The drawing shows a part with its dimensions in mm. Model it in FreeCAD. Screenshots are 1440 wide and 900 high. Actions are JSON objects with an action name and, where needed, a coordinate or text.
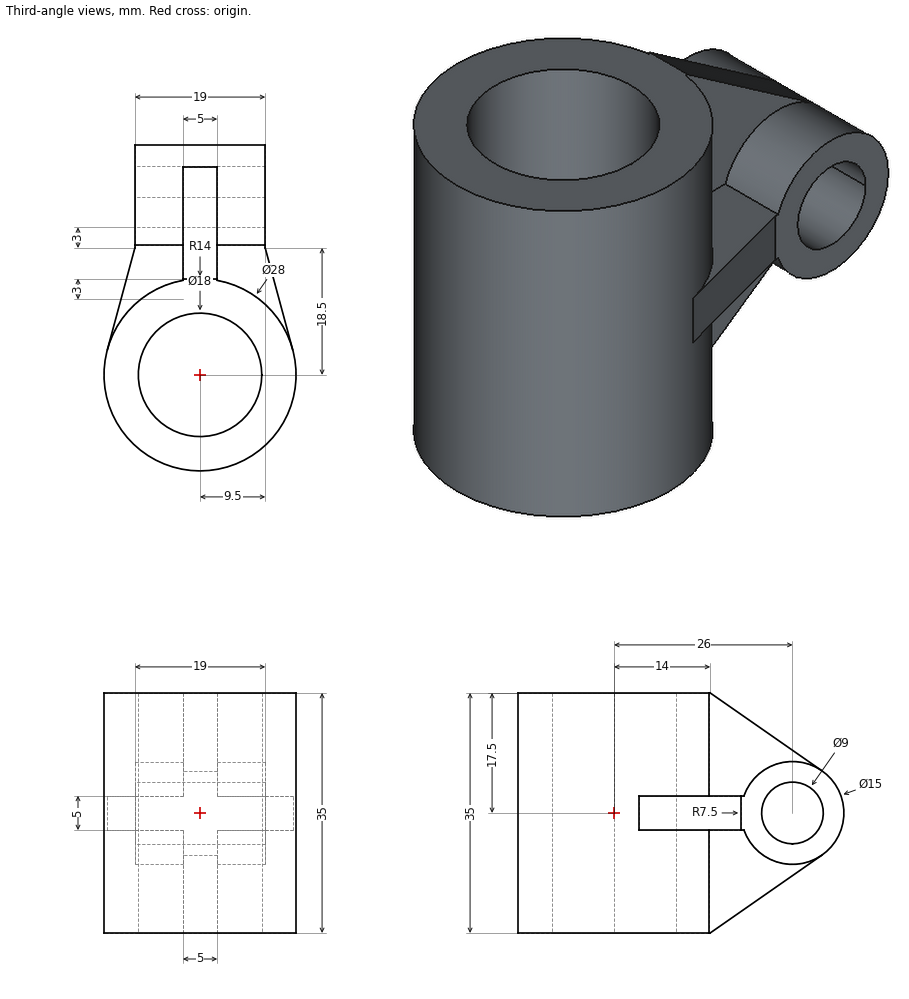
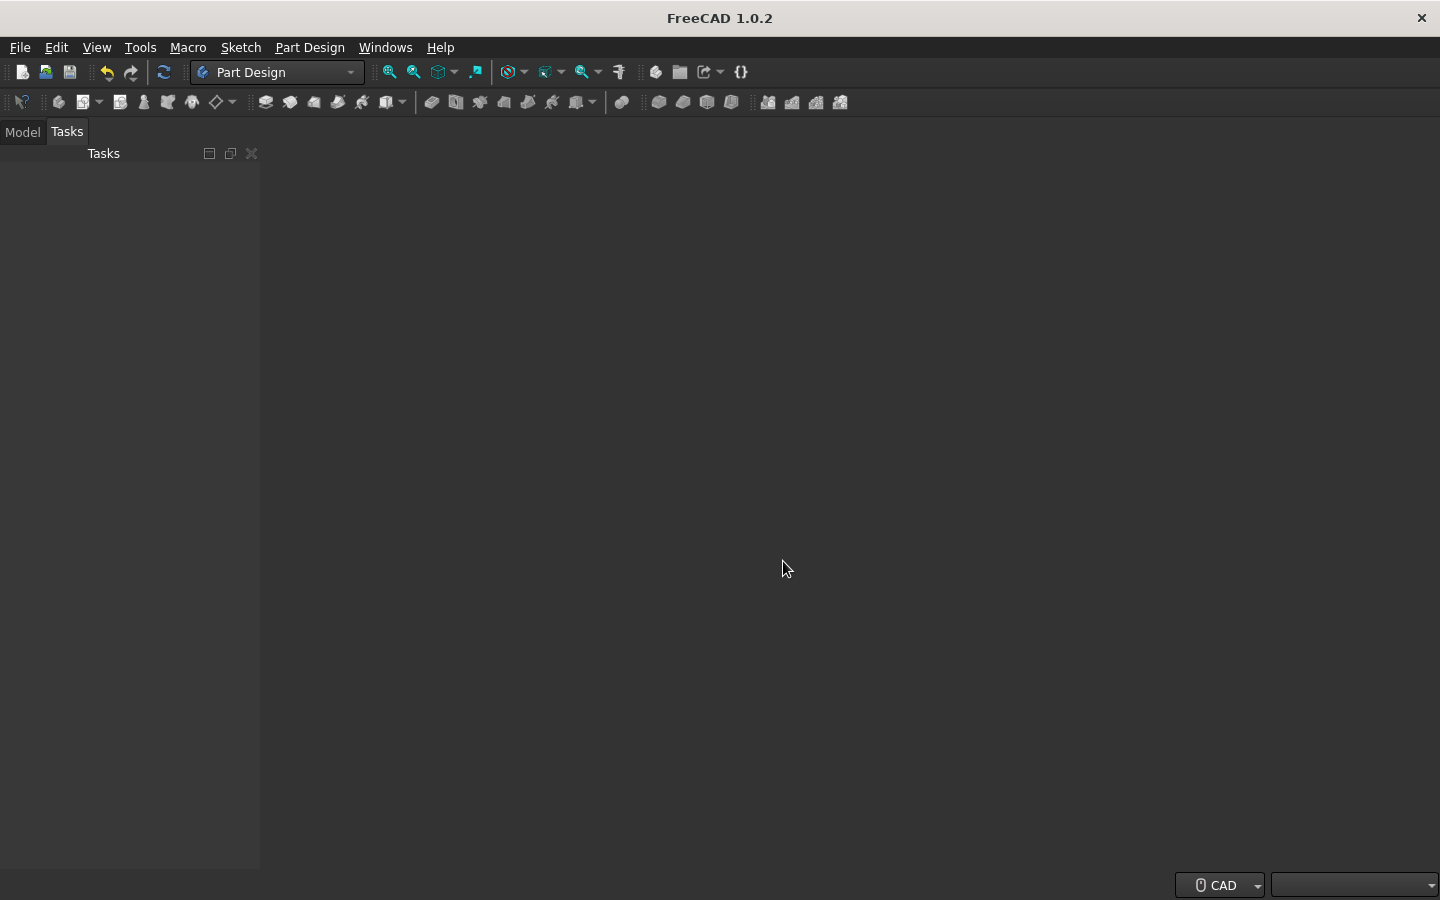
{"action": "key", "text": "ctrl+n"}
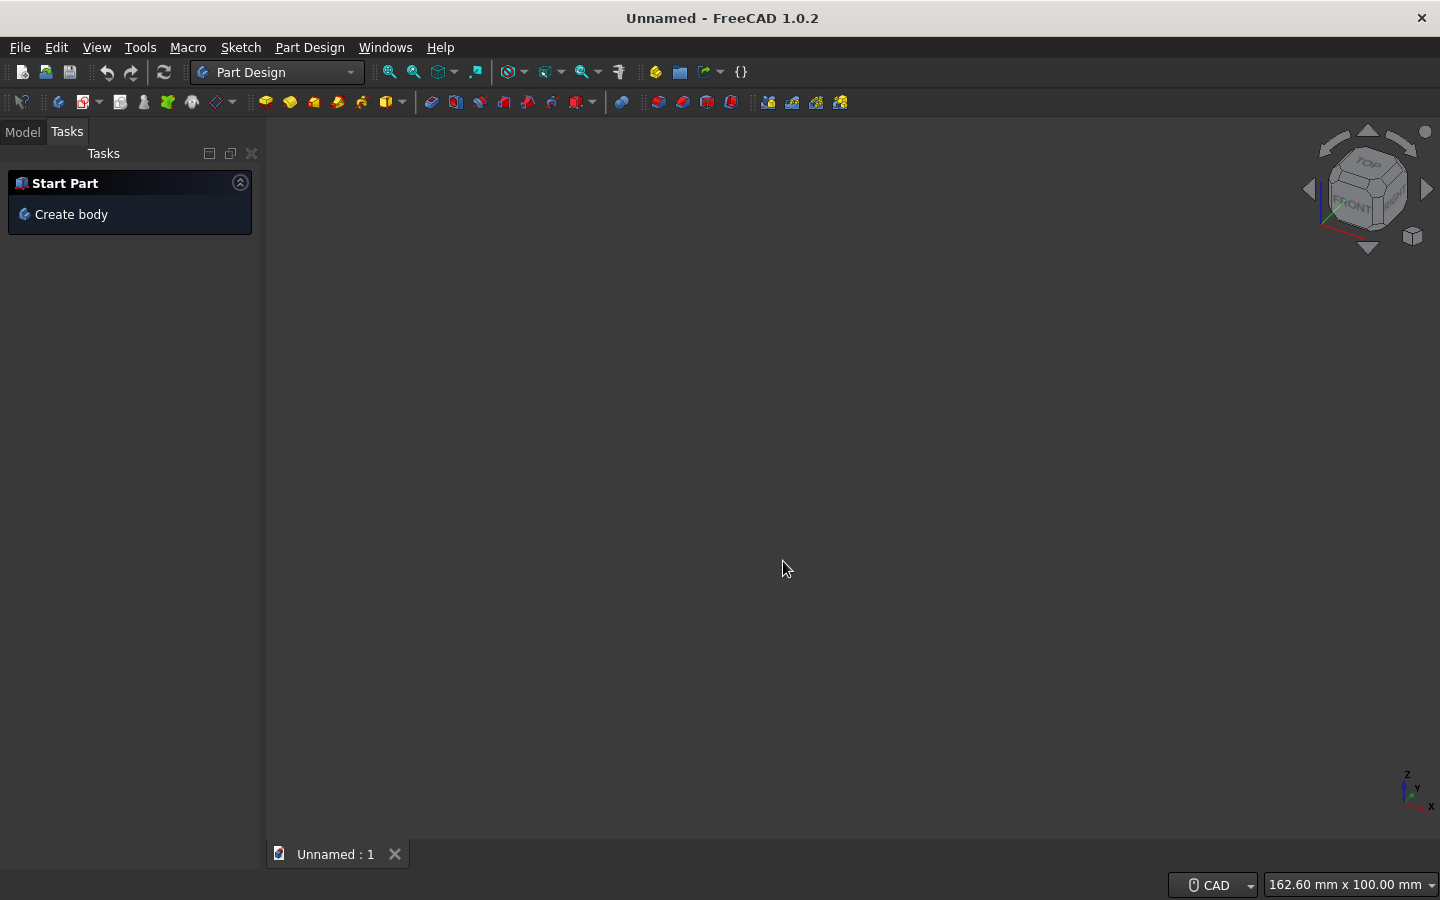
{"action": "left_click", "coordinate": [84, 102]}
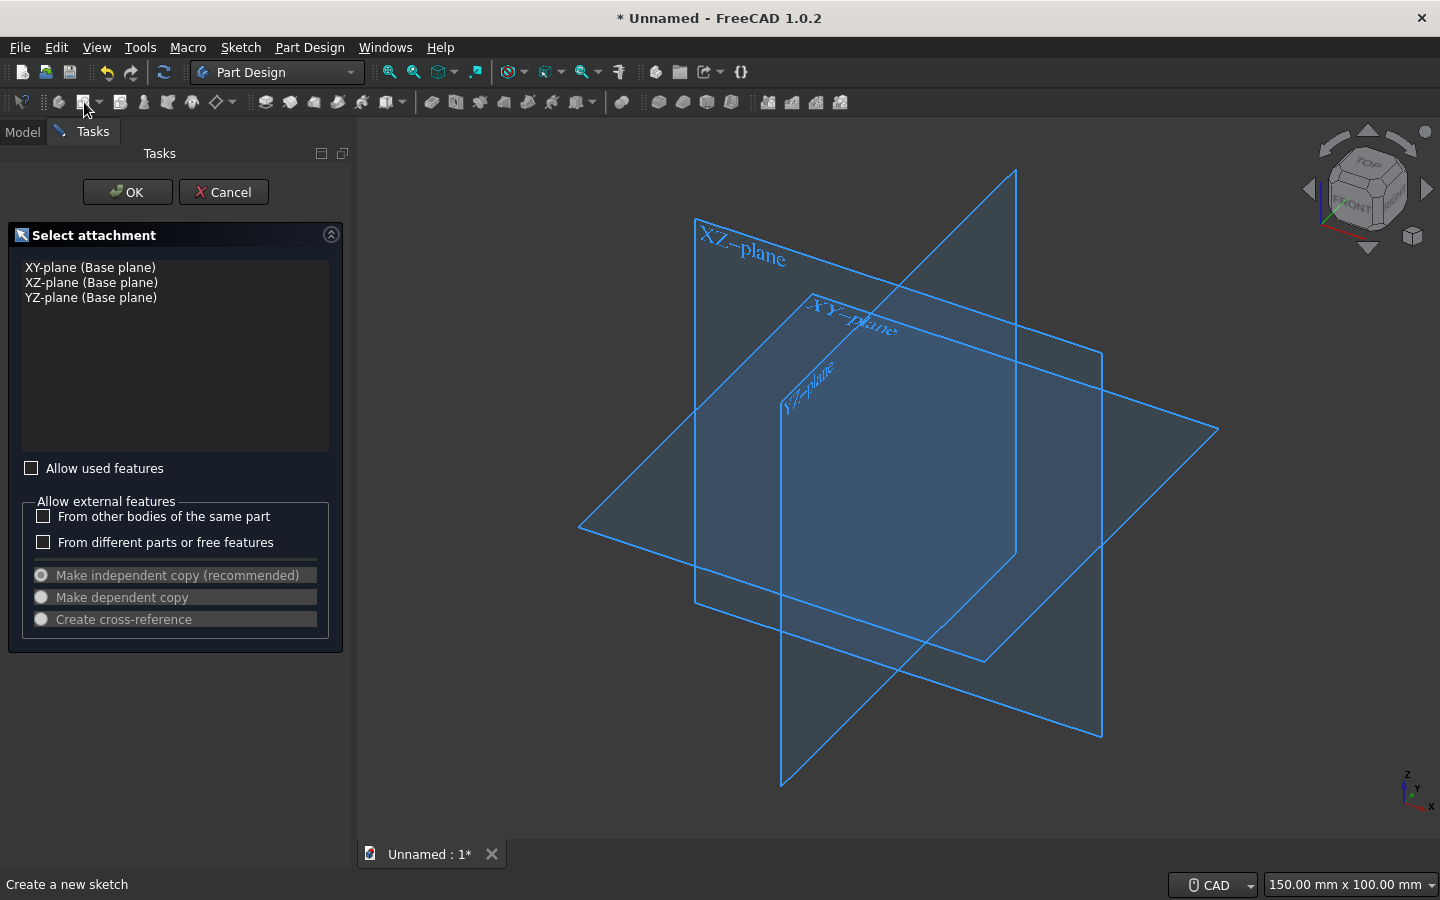
{"action": "left_click", "coordinate": [82, 268]}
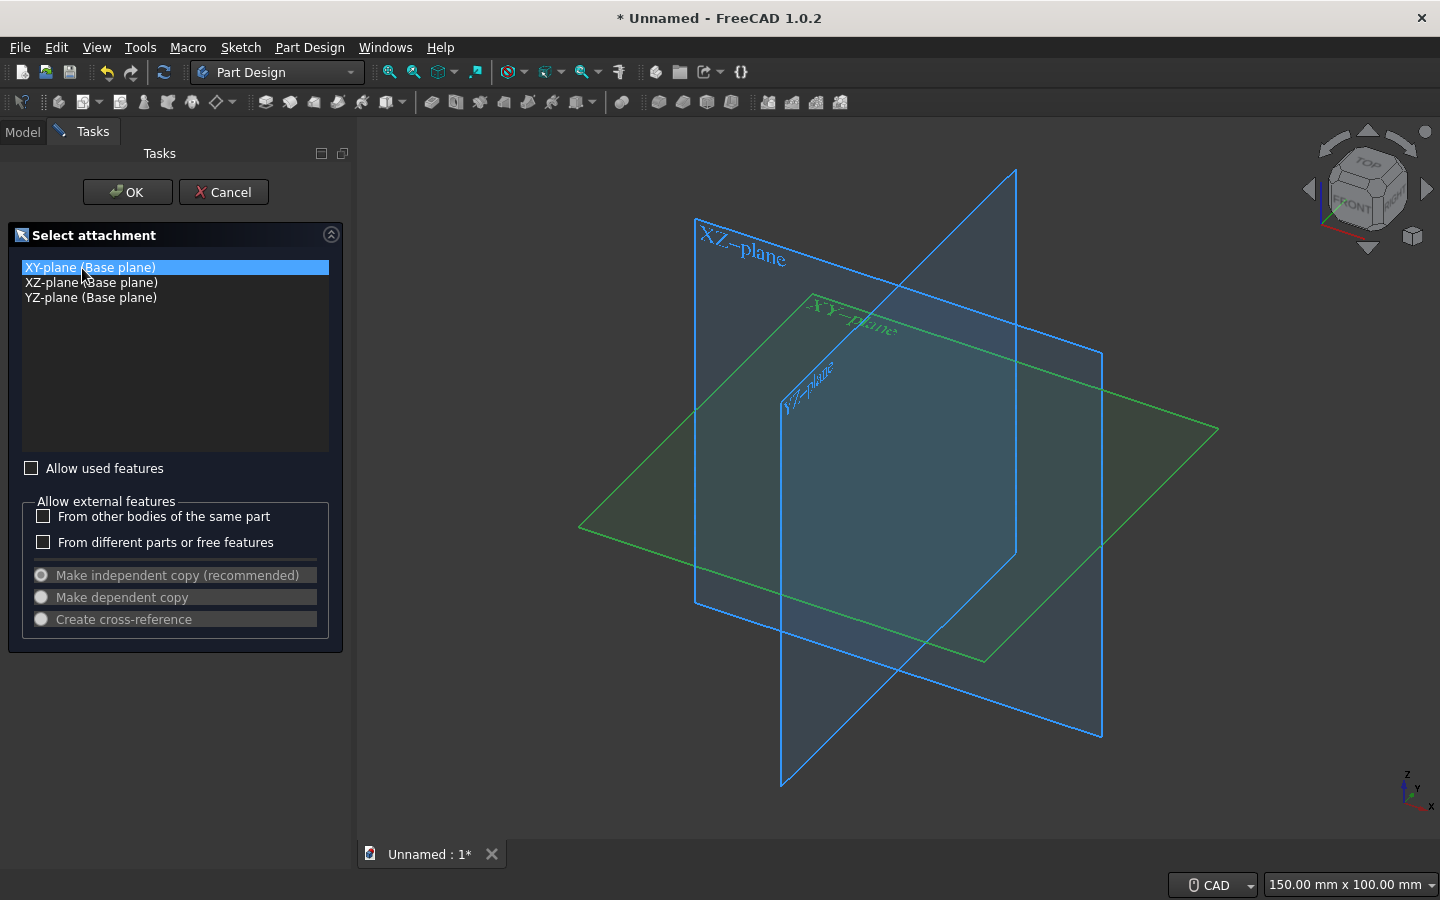
{"action": "left_click", "coordinate": [128, 192]}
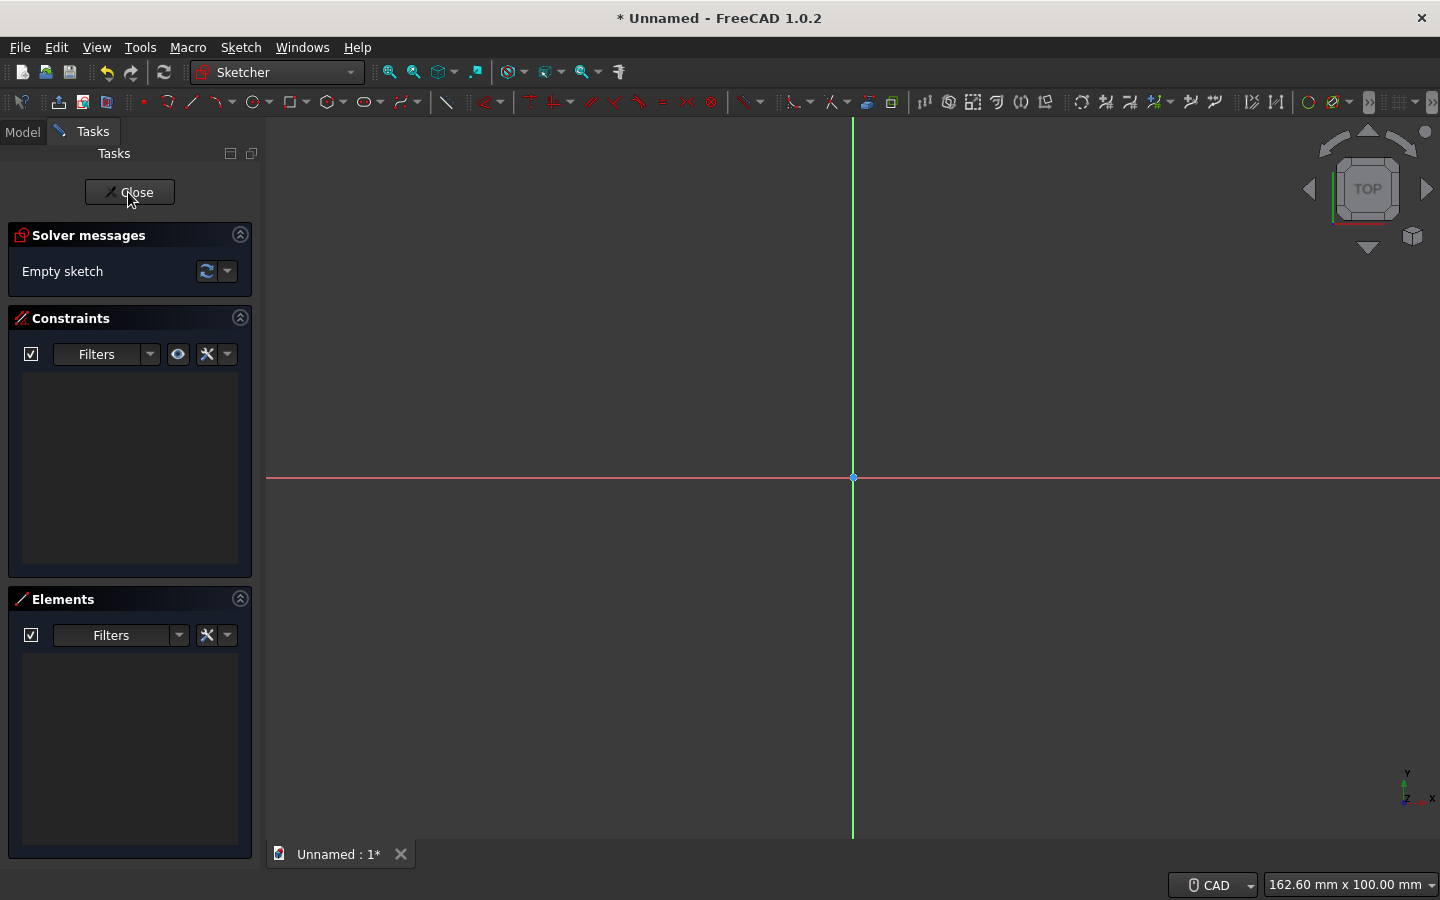
{"action": "scroll", "coordinate": [909, 478], "scroll_direction": "up", "scroll_amount": 4}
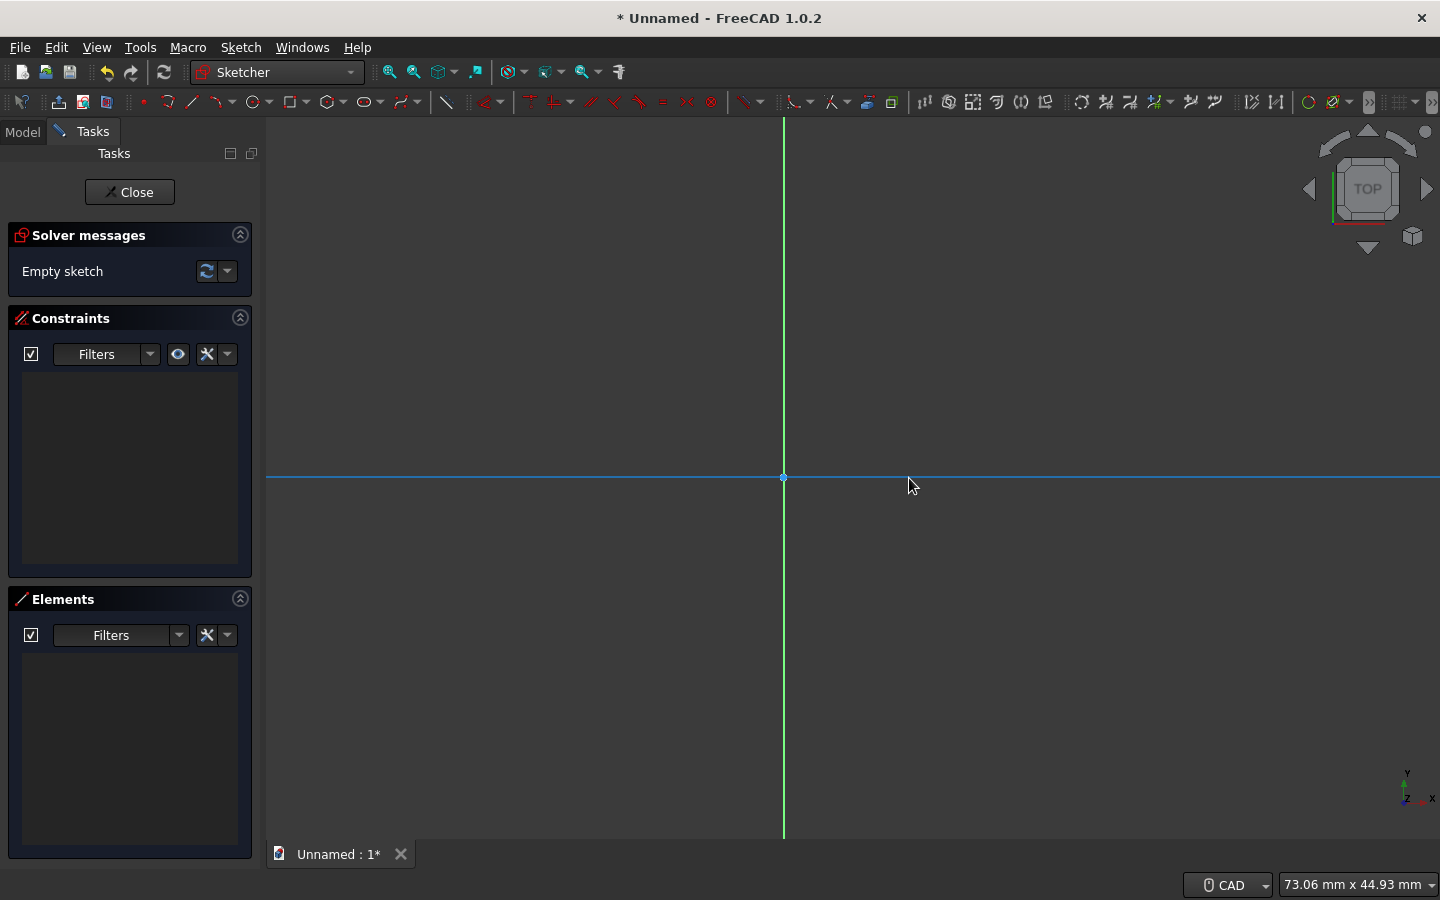
{"action": "key", "text": "g c"}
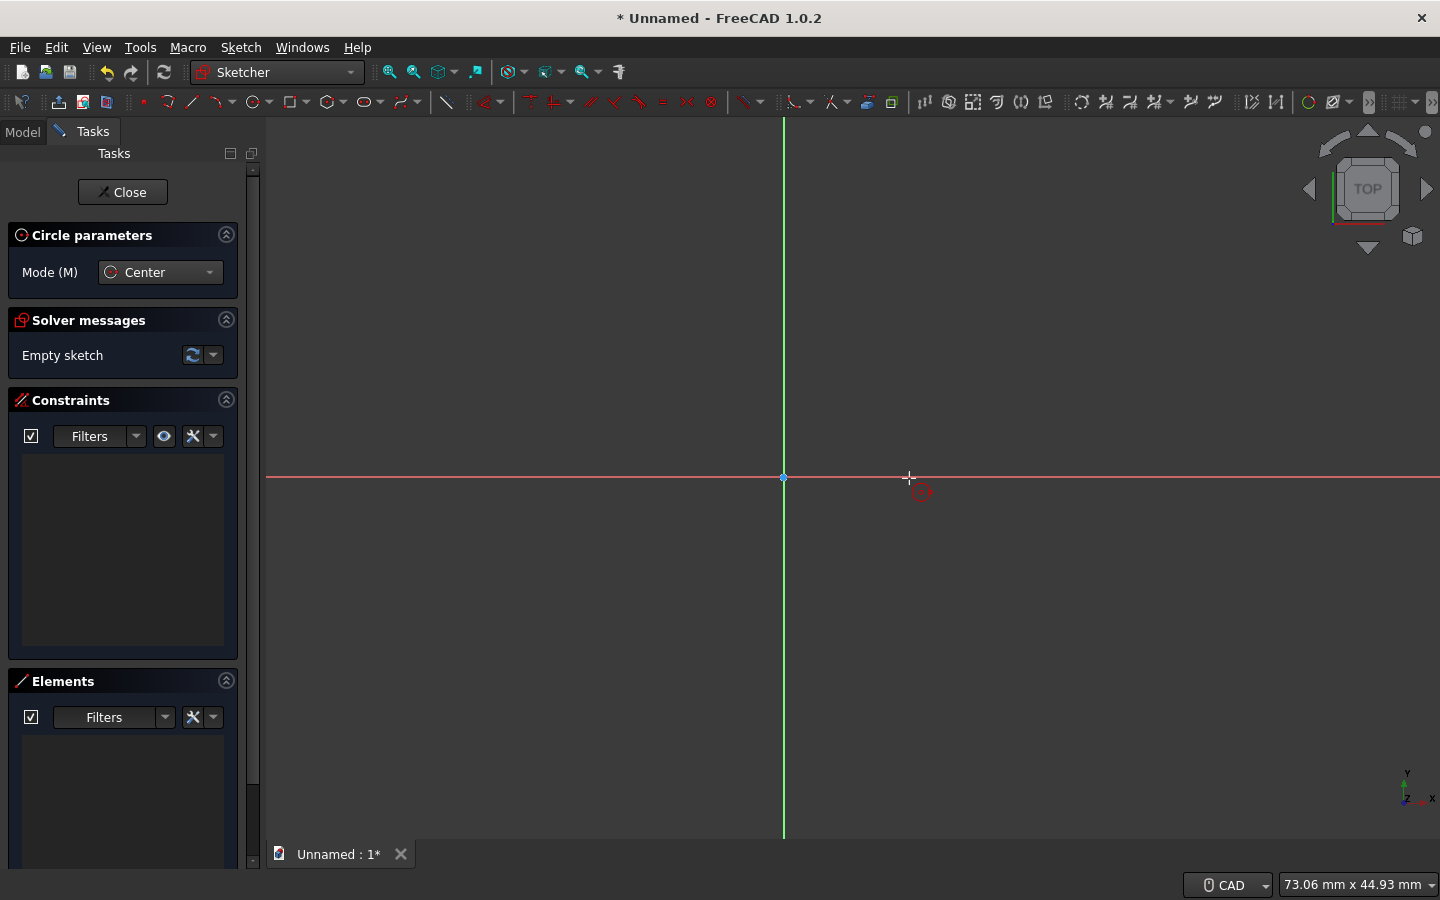
{"action": "left_click", "coordinate": [784, 477]}
{"action": "left_click", "coordinate": [943, 318]}